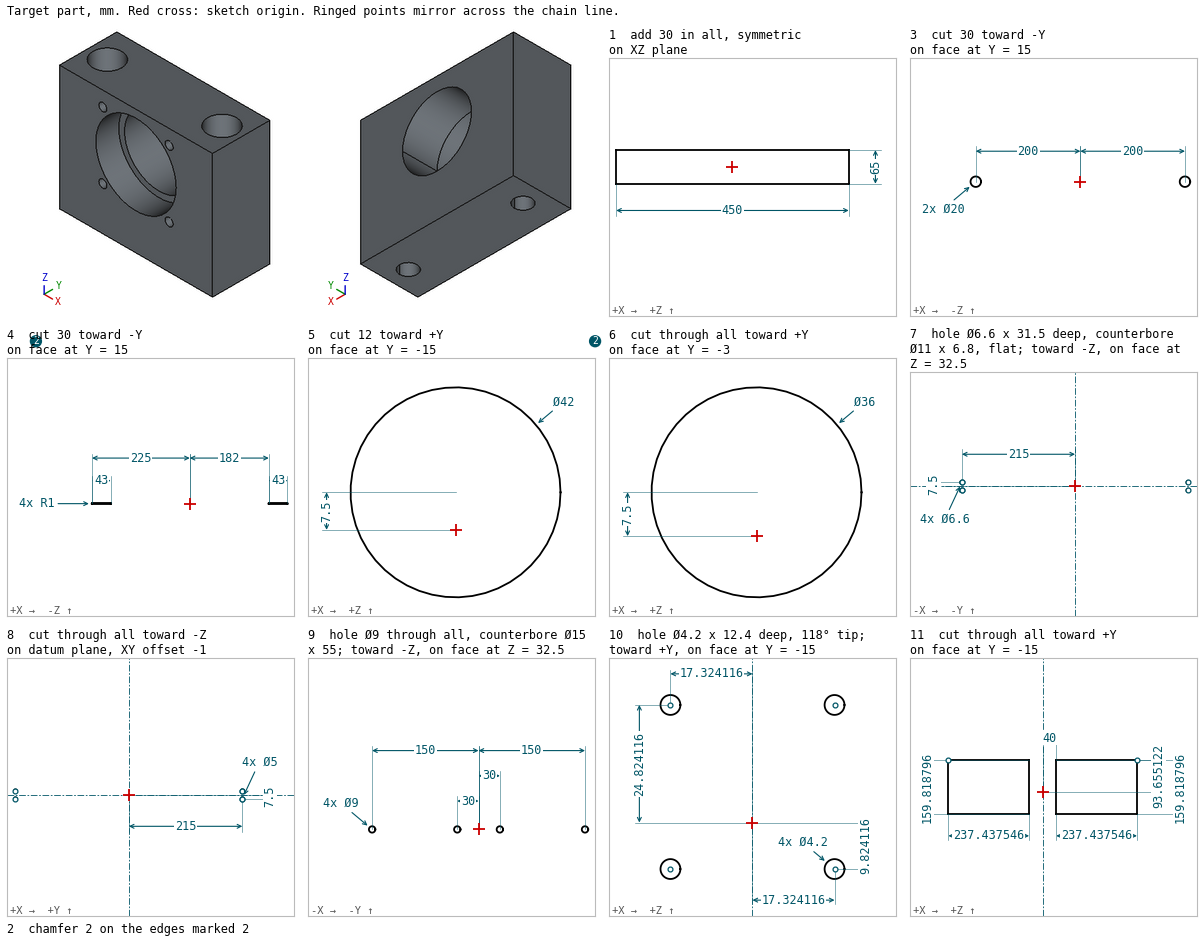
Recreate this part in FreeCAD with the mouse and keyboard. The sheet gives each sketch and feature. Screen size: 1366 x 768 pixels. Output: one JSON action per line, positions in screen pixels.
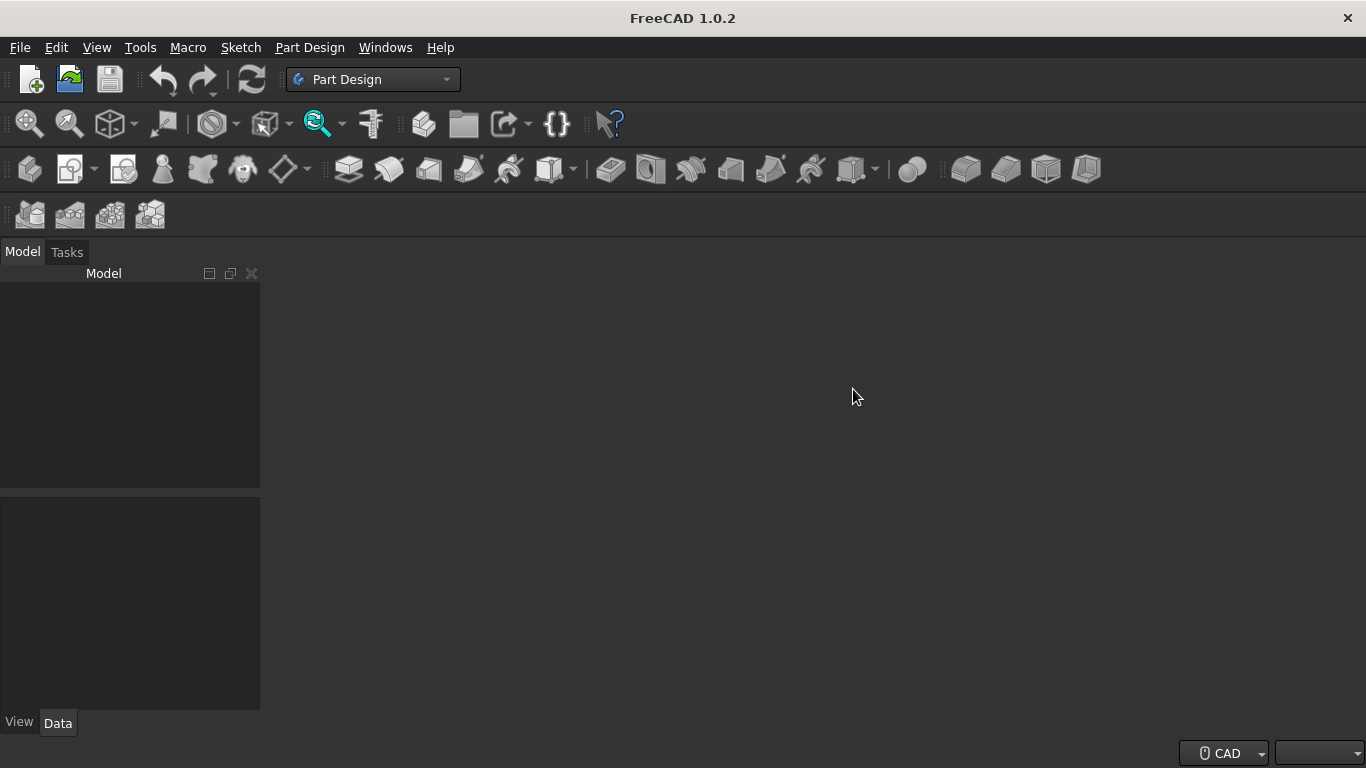
{"action": "key", "text": "ctrl+n"}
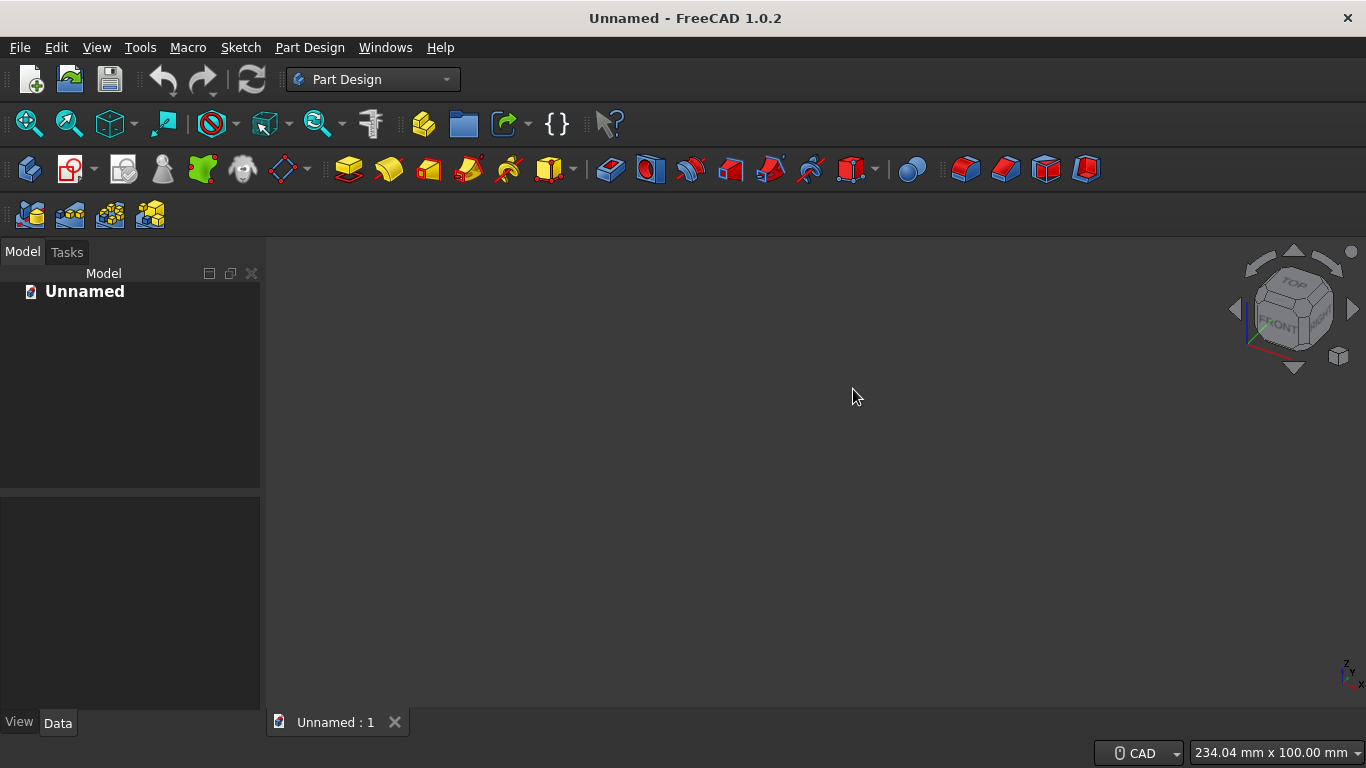
{"action": "left_click", "coordinate": [70, 170]}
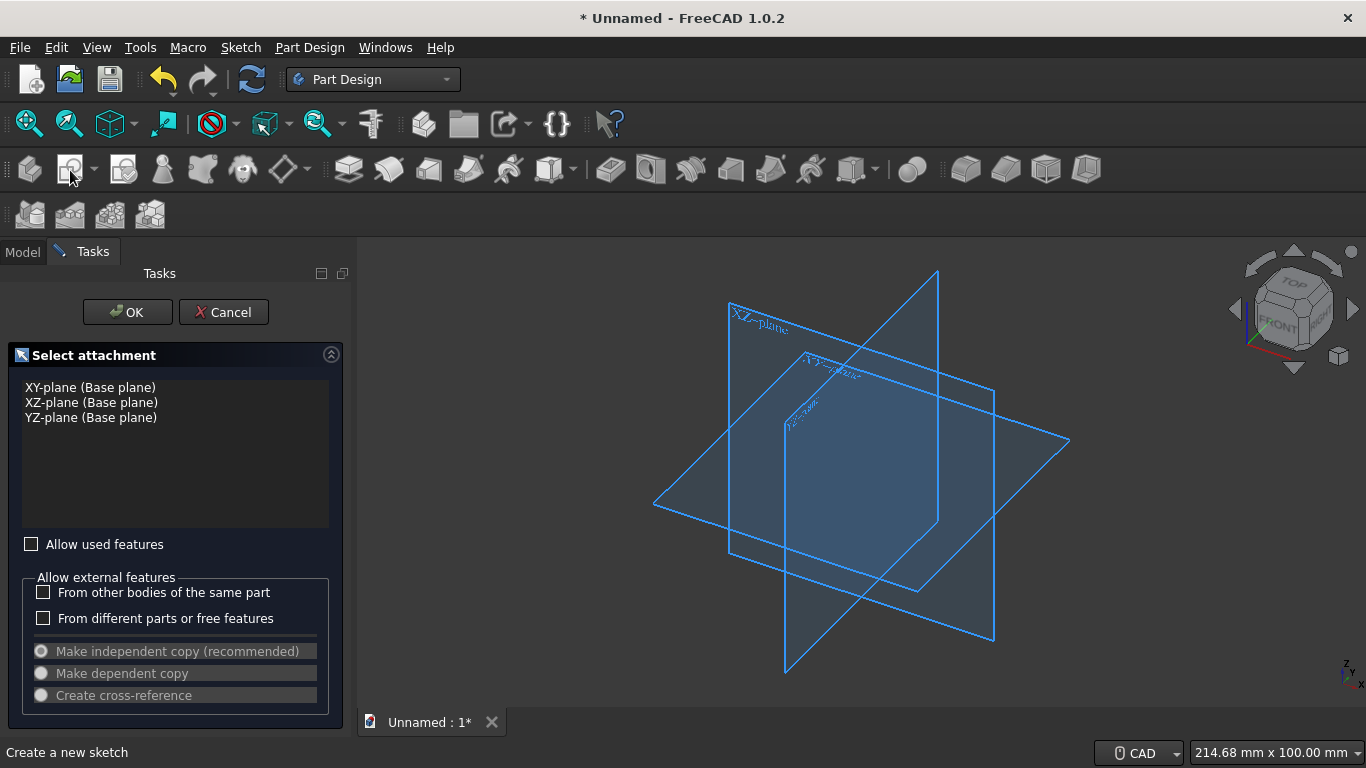
{"action": "left_click", "coordinate": [82, 402]}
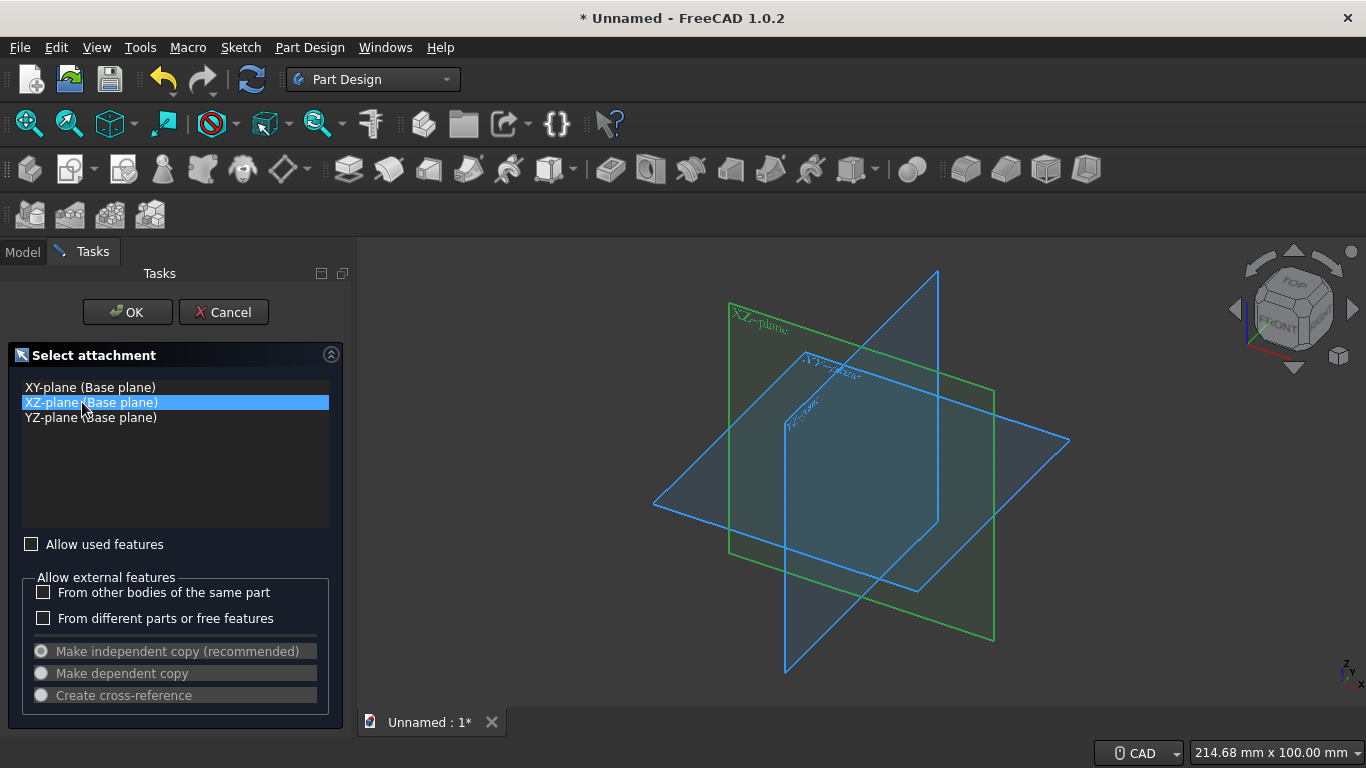
{"action": "left_click", "coordinate": [128, 312]}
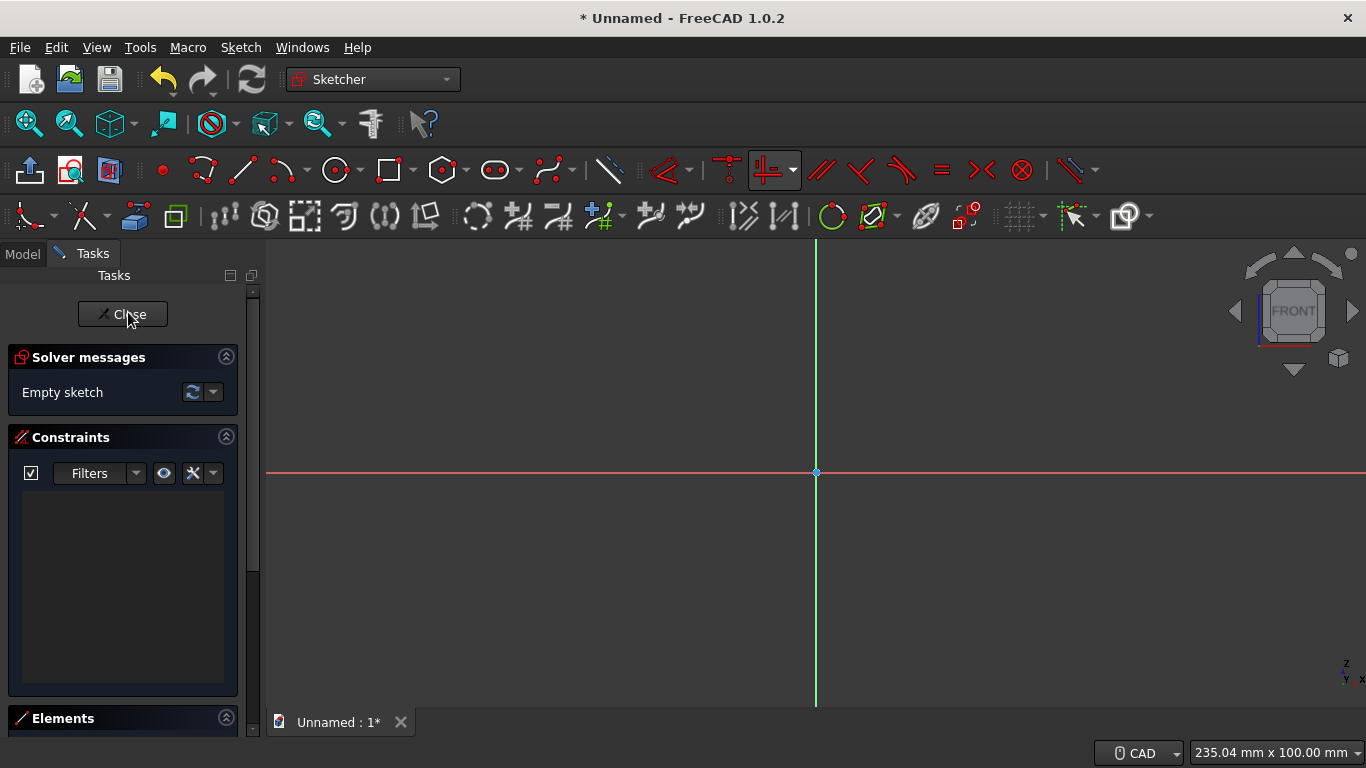
{"action": "scroll", "coordinate": [718, 473], "scroll_direction": "down", "scroll_amount": 6}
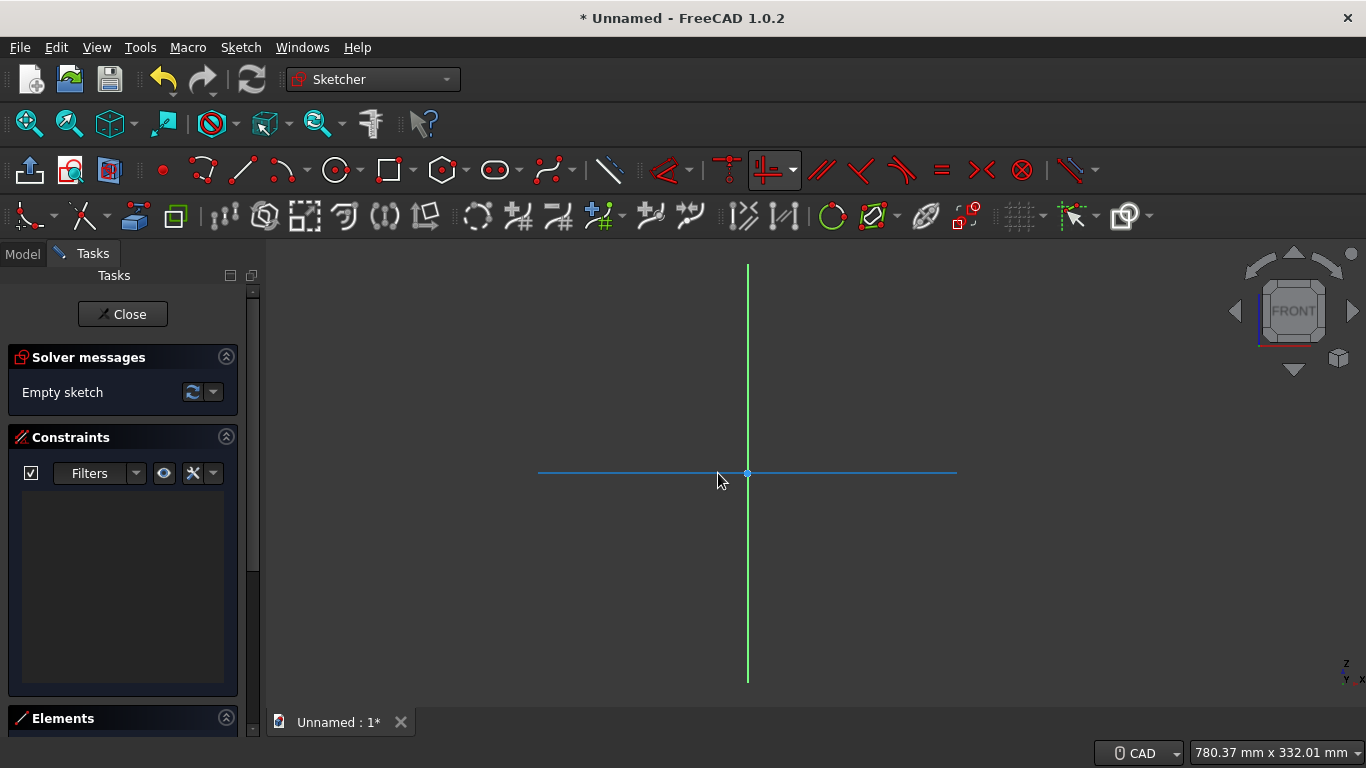
{"action": "key", "text": "g v"}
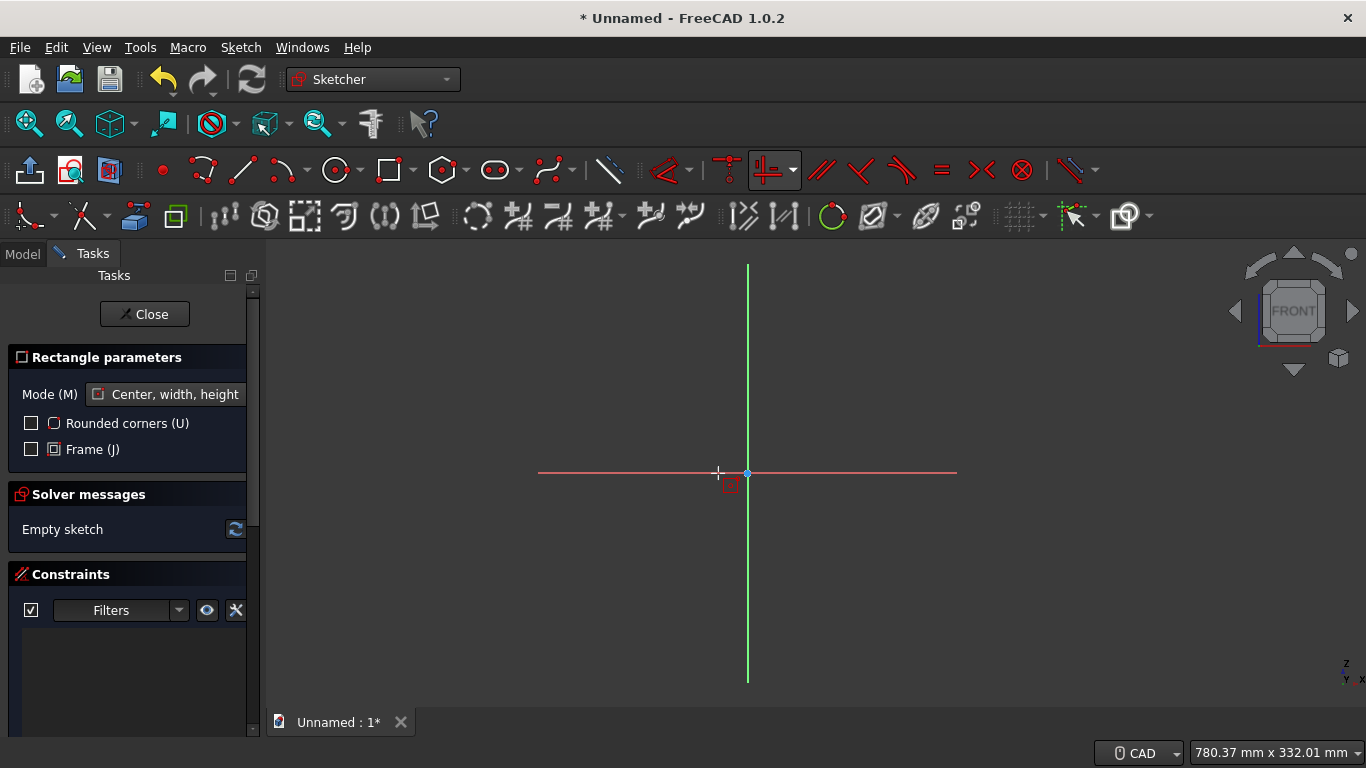
{"action": "left_click", "coordinate": [748, 473]}
{"action": "mouse_move", "coordinate": [1065, 428]}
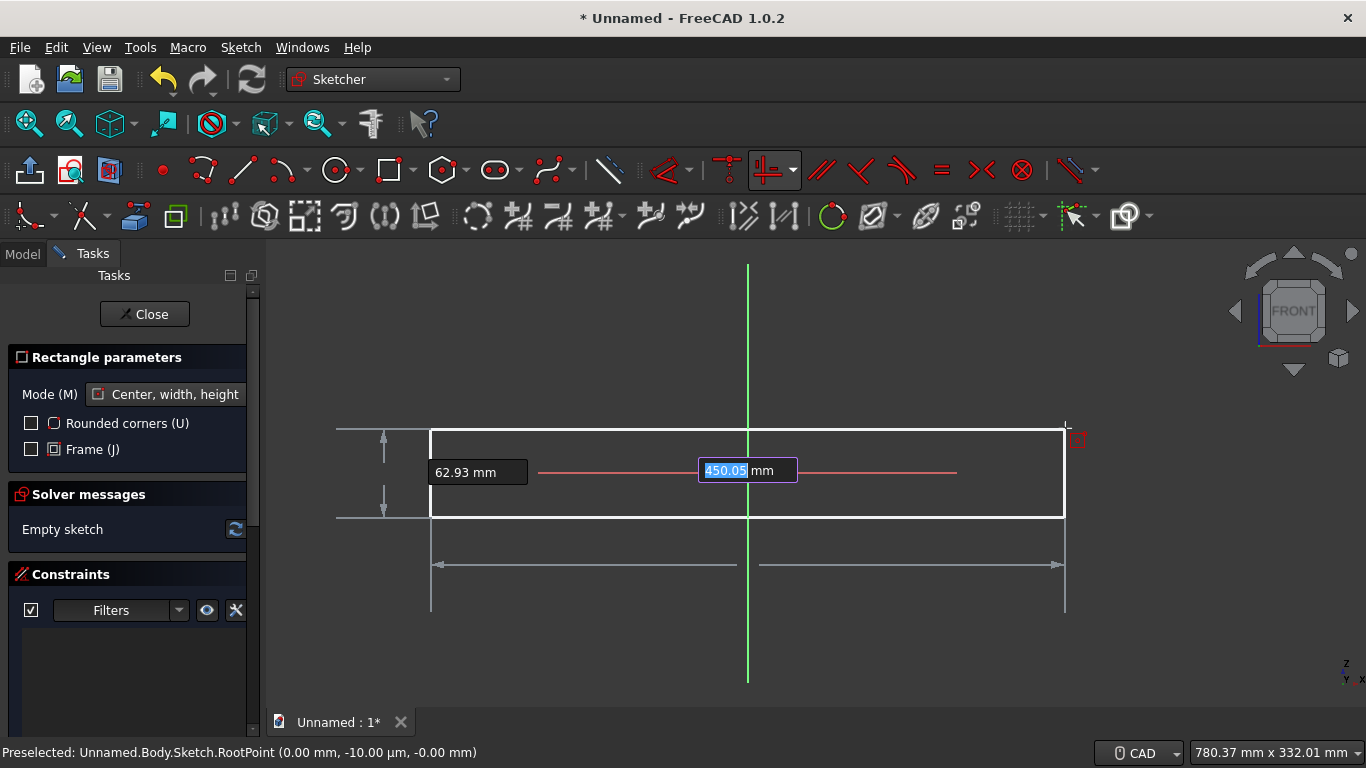
{"action": "type", "text": "450"}
{"action": "key", "text": "Tab"}
{"action": "type", "text": "65"}
{"action": "key", "text": "Return"}
{"action": "key", "text": "Escape"}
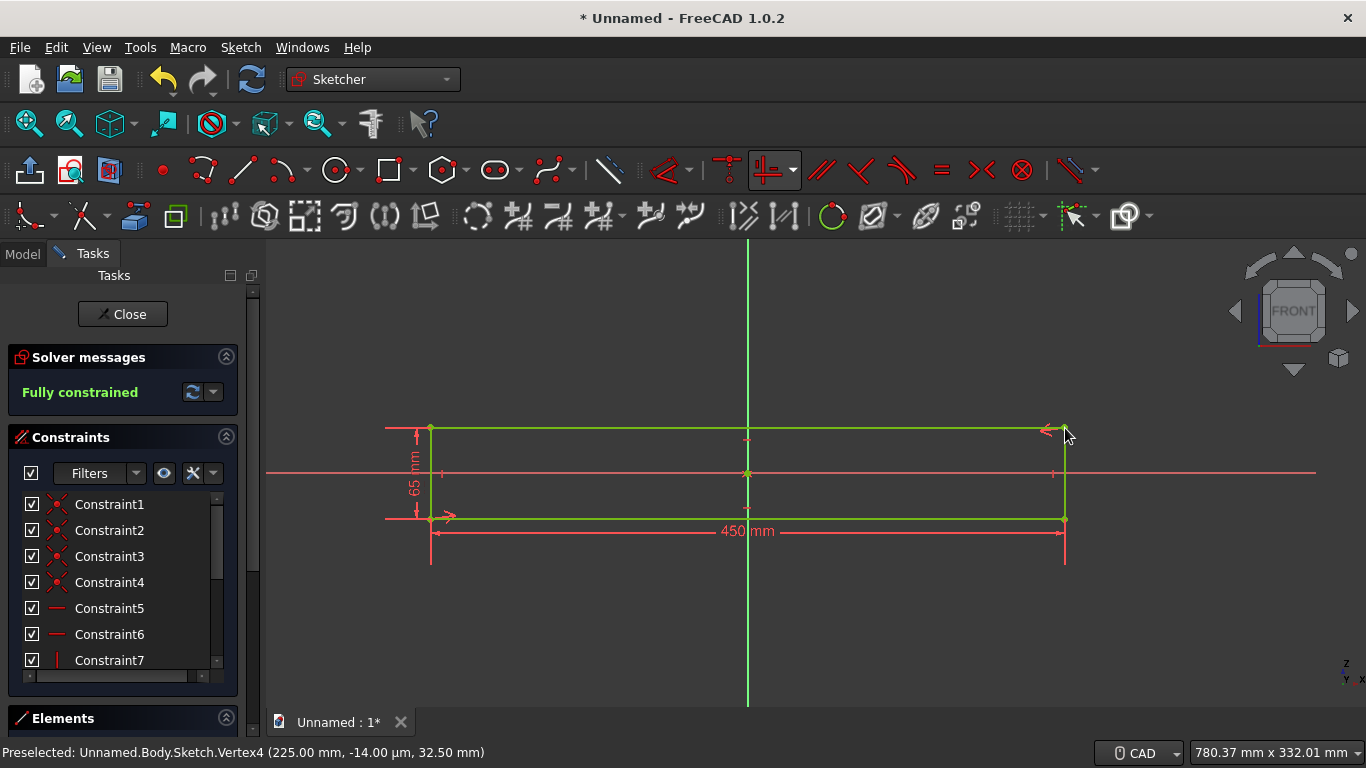
{"action": "left_click", "coordinate": [123, 314]}